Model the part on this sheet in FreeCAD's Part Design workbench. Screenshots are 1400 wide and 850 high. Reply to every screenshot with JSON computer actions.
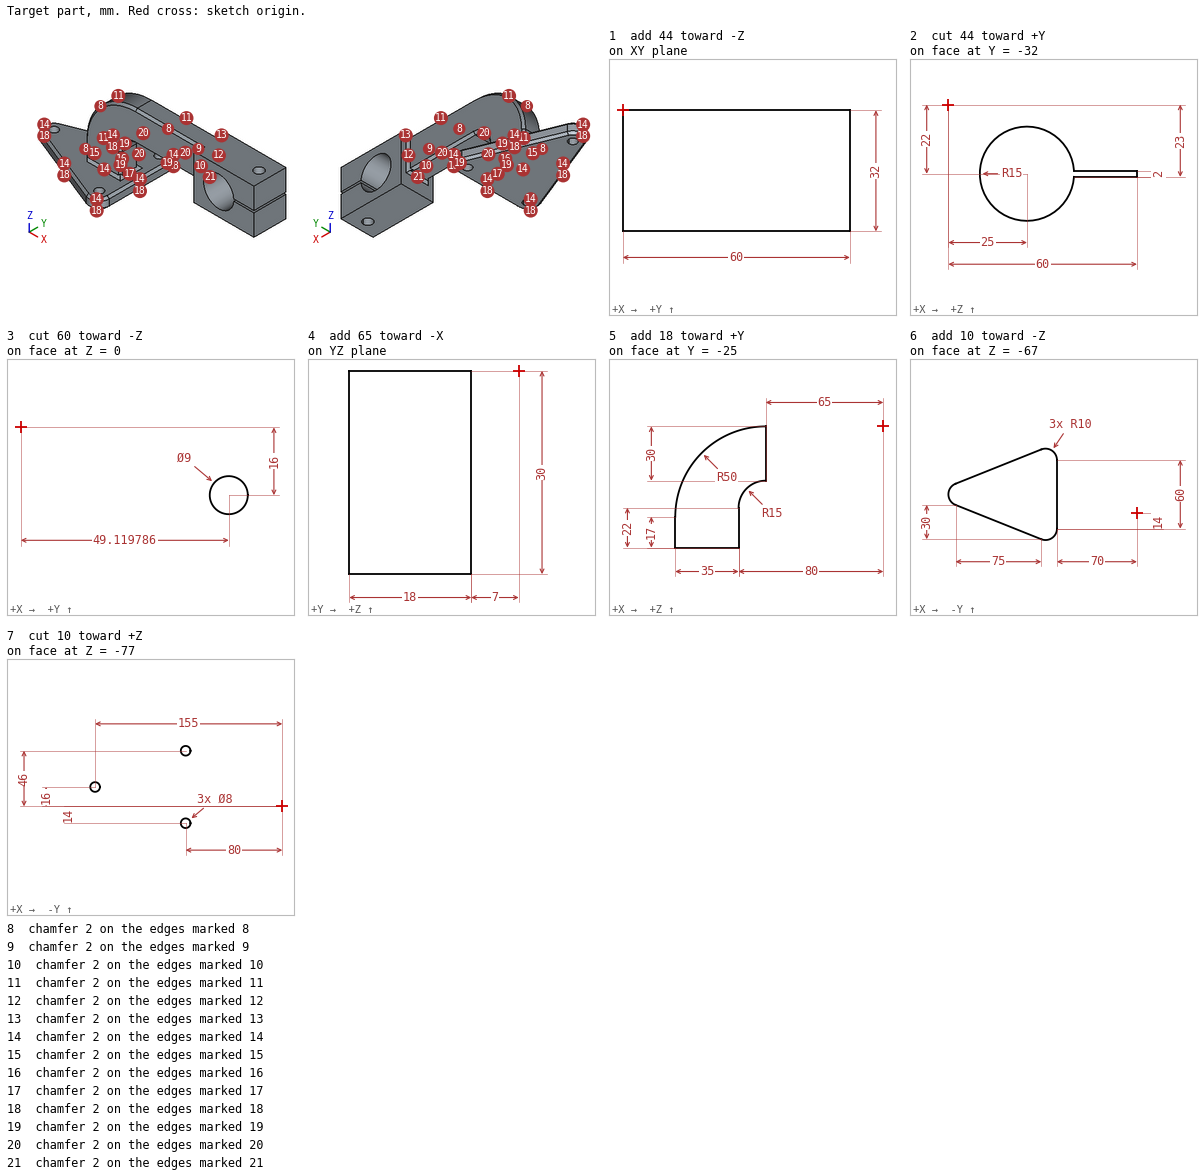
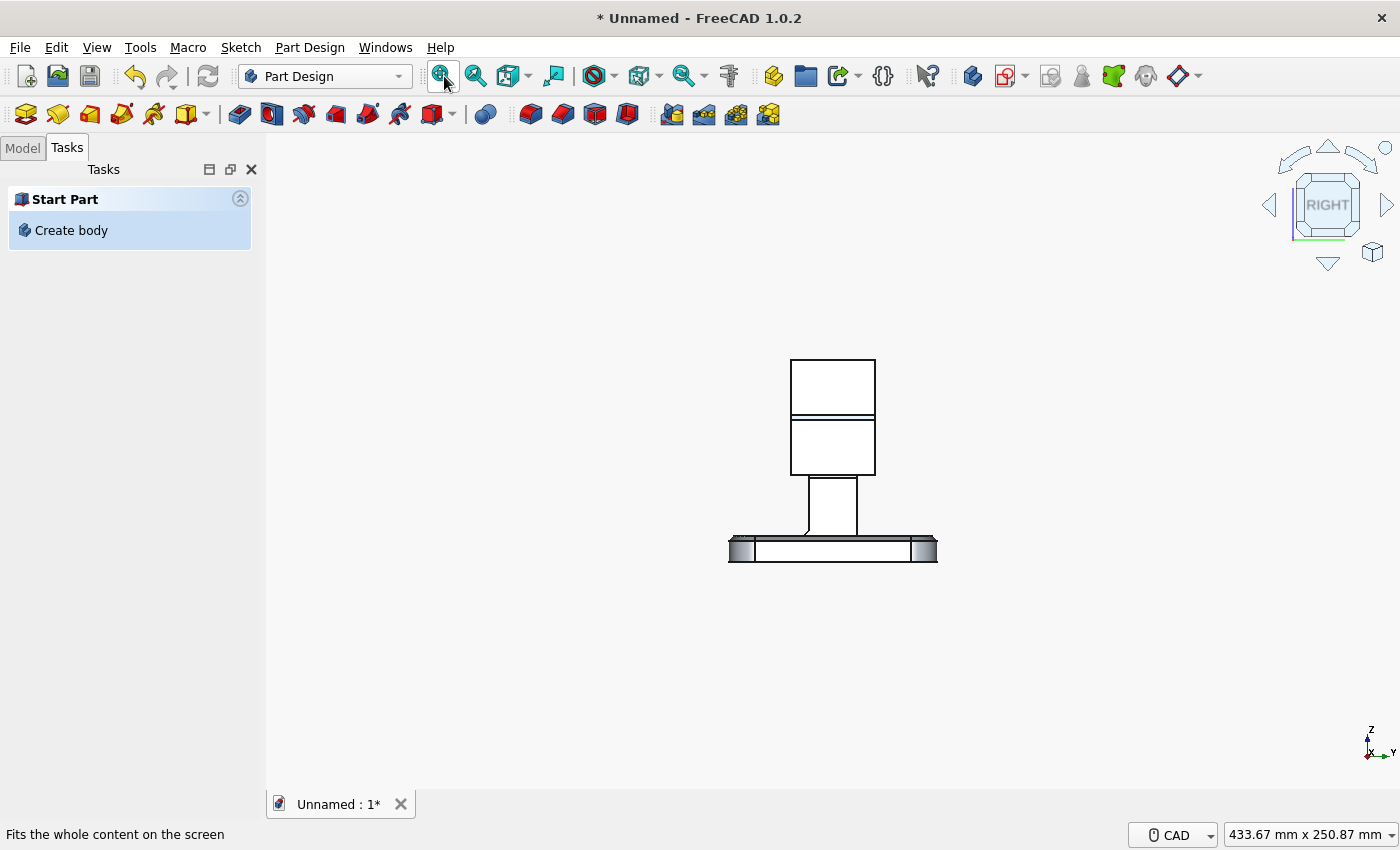
{"action": "key", "text": "5"}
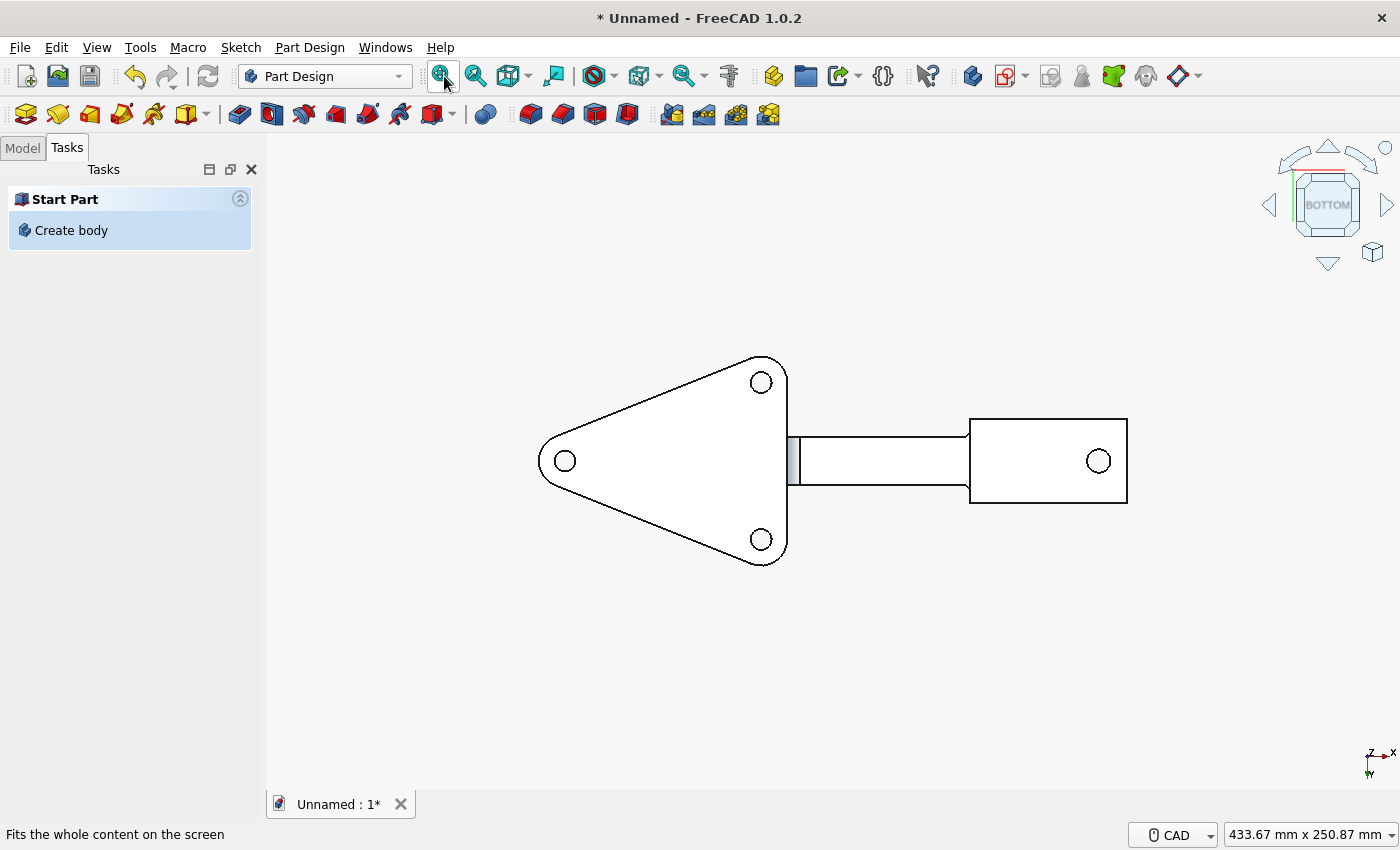
{"action": "key", "text": "4"}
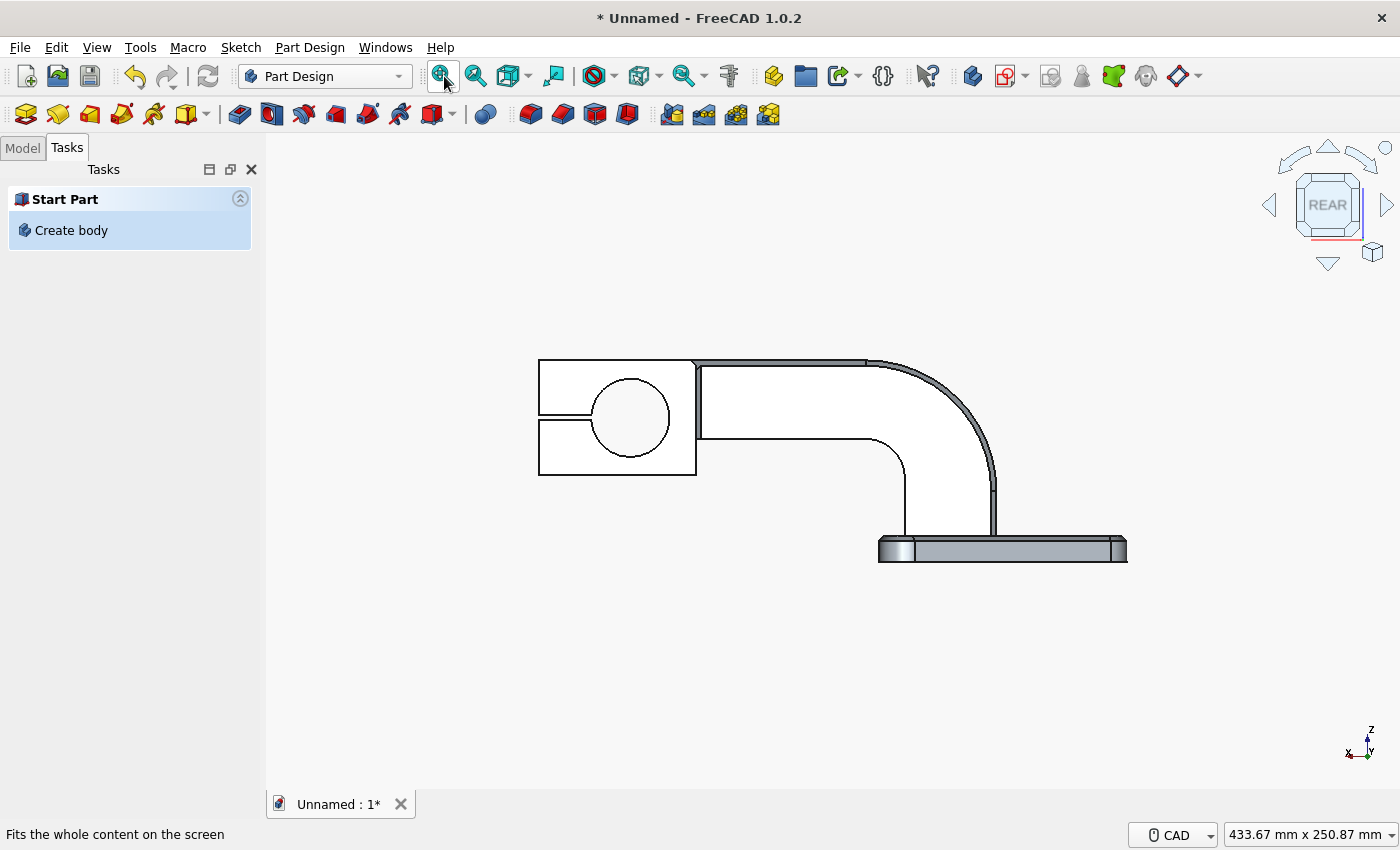
{"action": "key", "text": "6"}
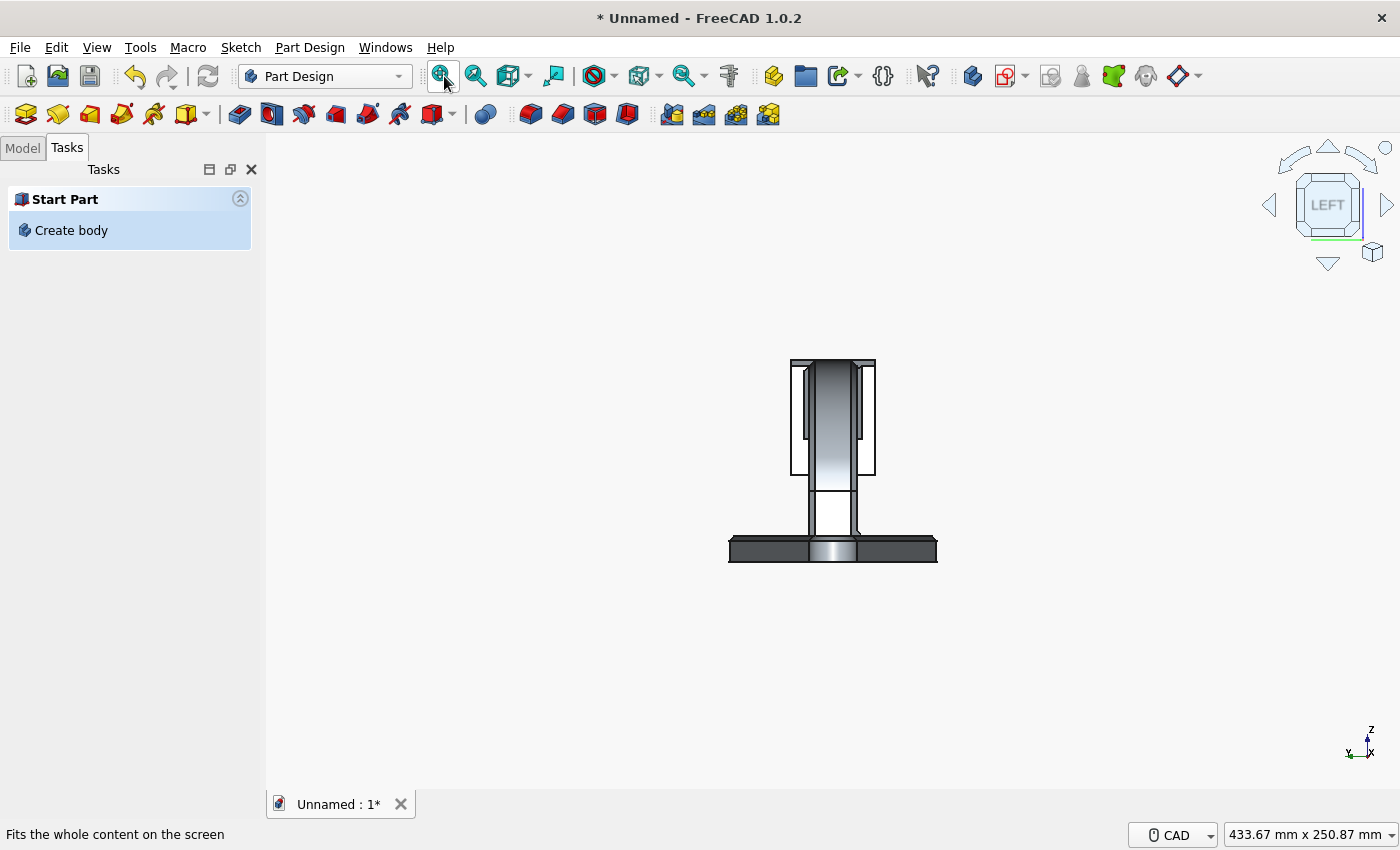
{"action": "left_click", "coordinate": [444, 76]}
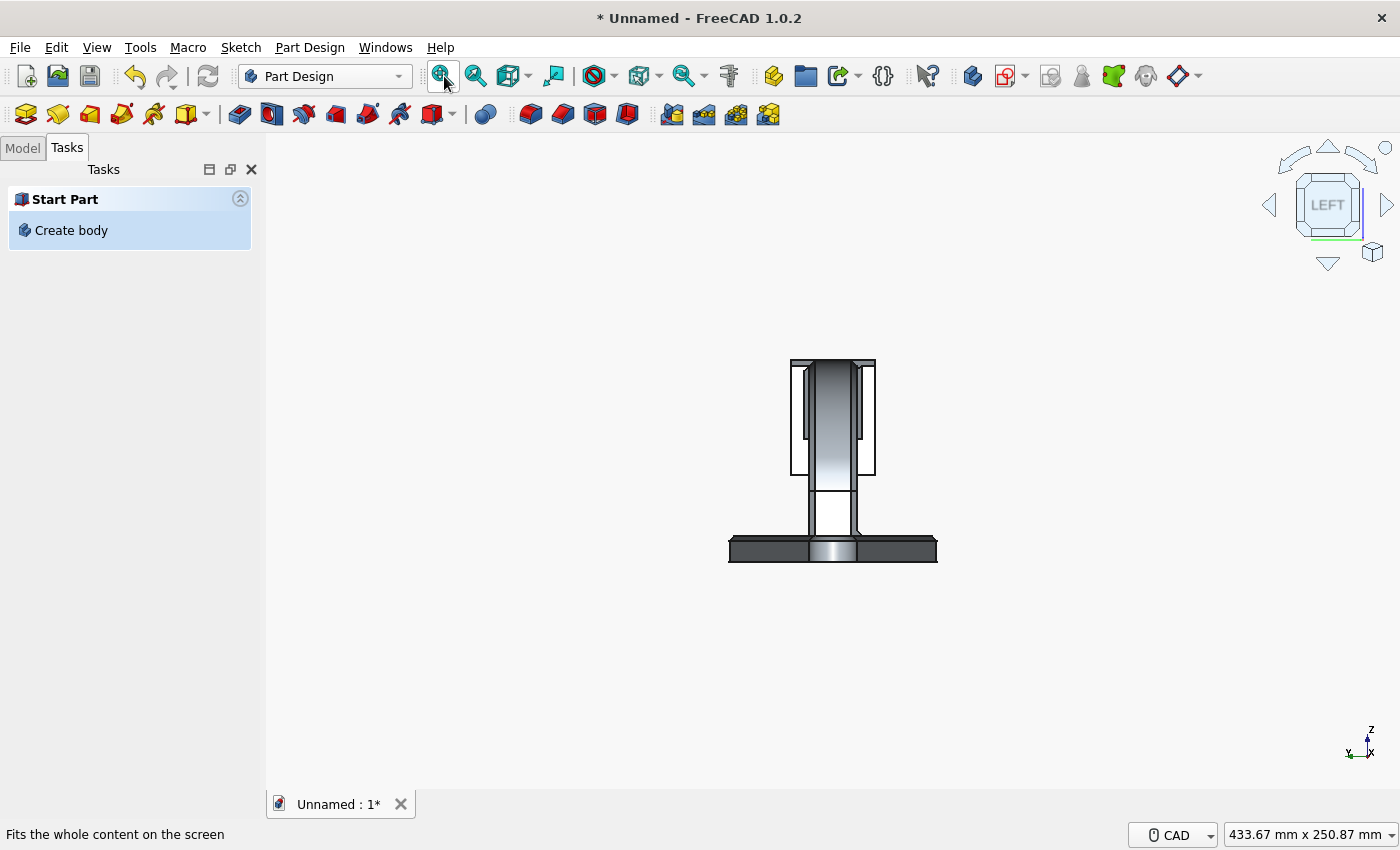
{"action": "key", "text": "v 3"}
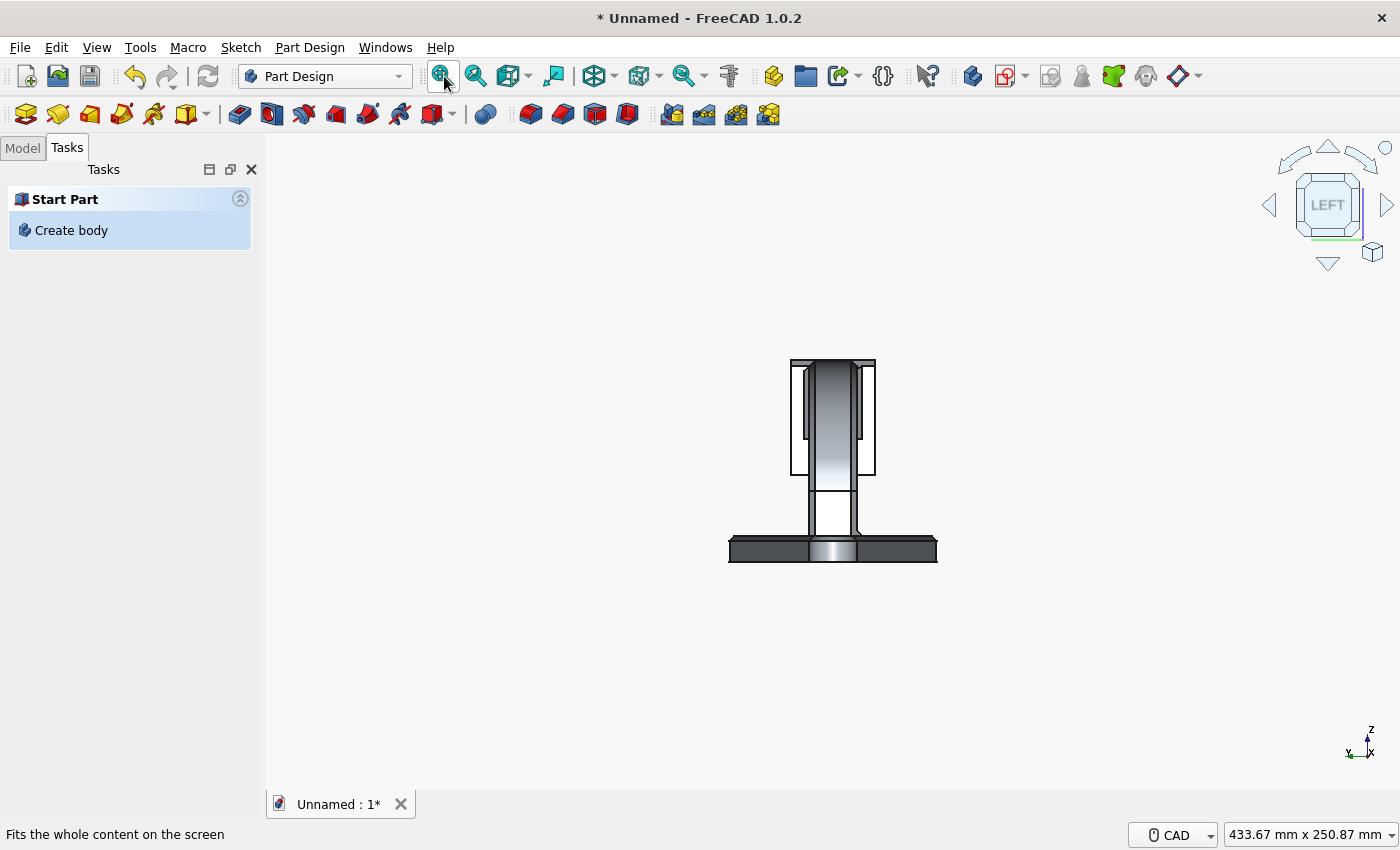
{"action": "key", "text": "0"}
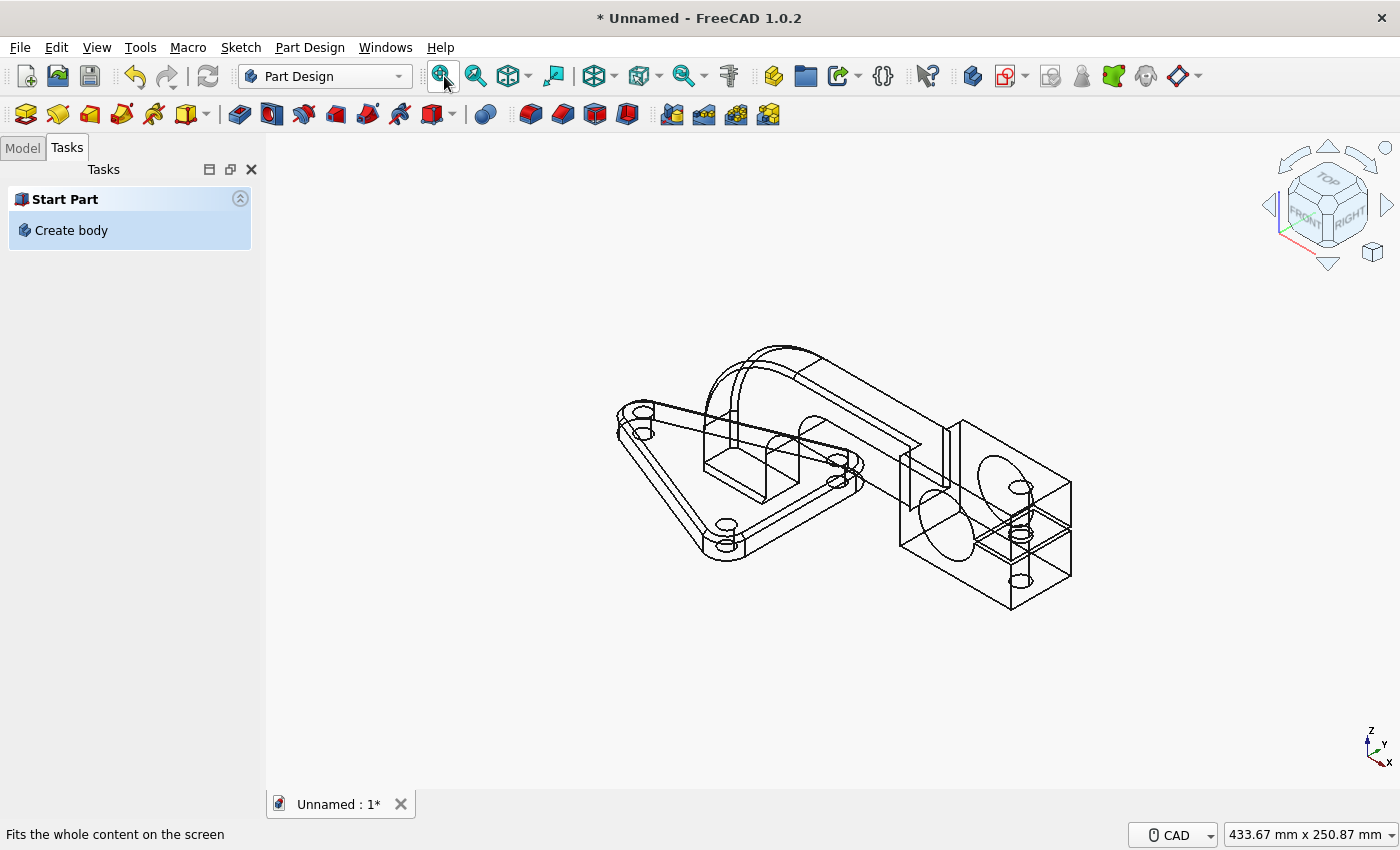
{"action": "left_click", "coordinate": [717, 454]}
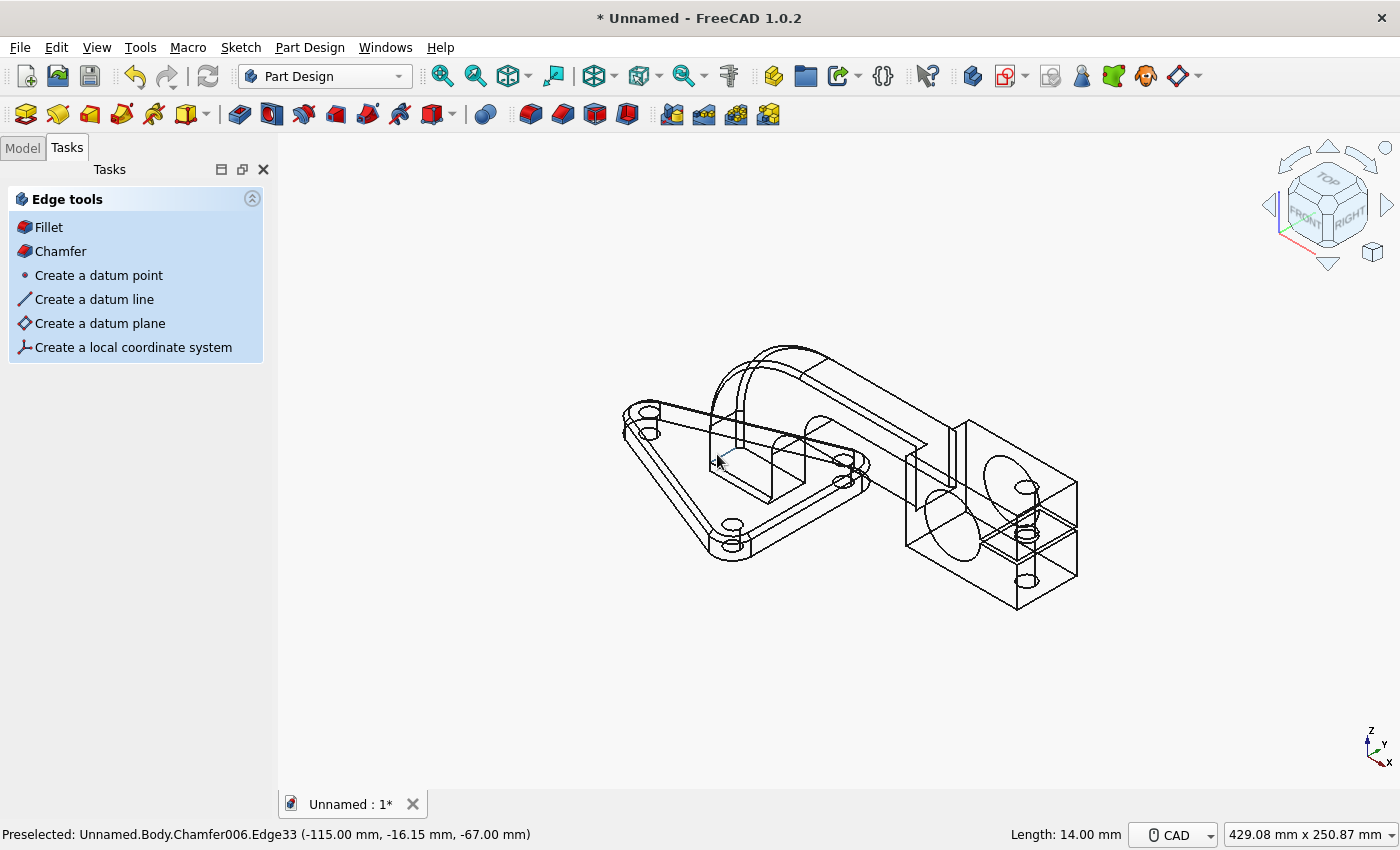
{"action": "key", "text": "v 1"}